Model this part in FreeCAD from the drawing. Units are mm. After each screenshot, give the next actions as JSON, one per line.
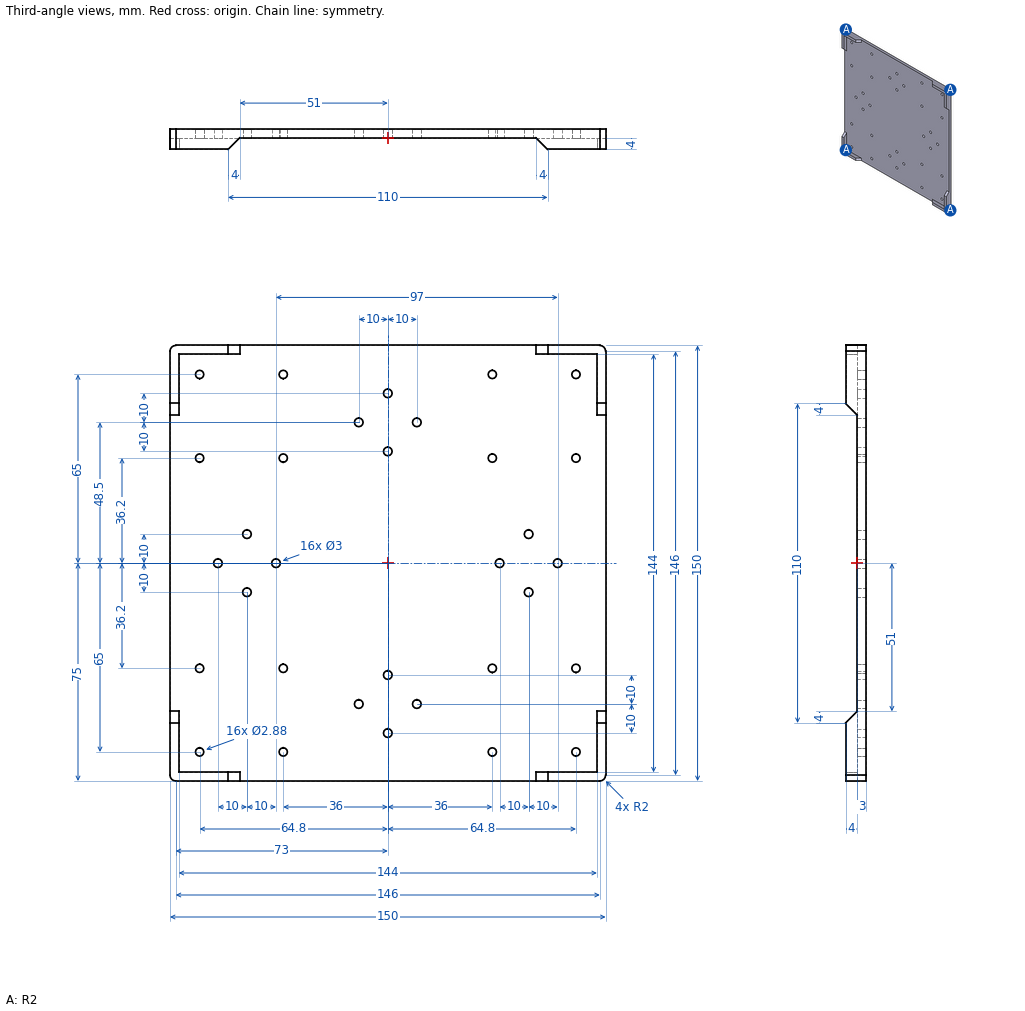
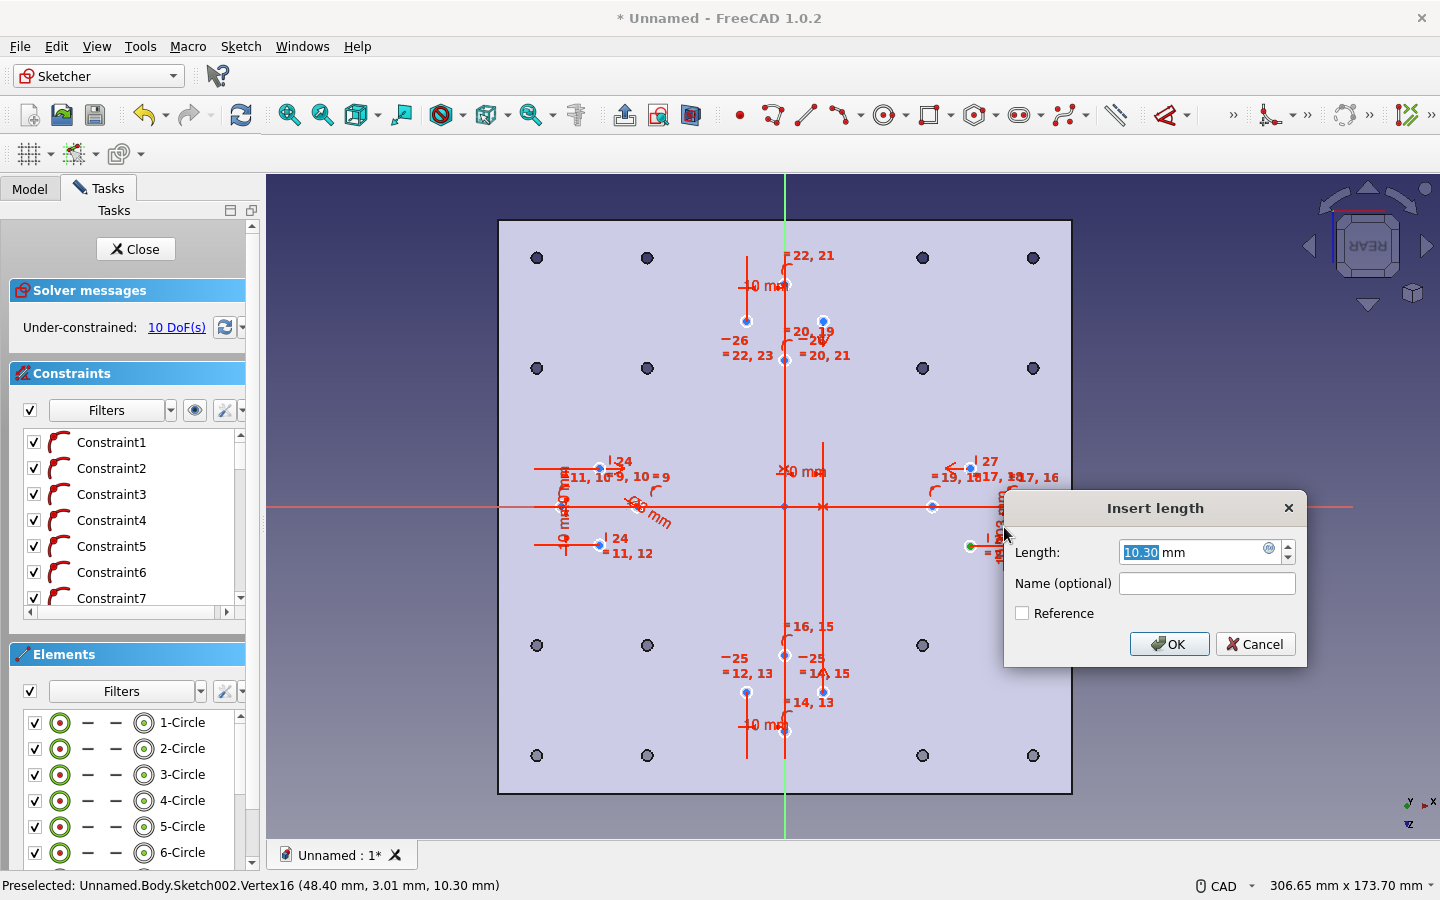
{"action": "type", "text": "10"}
{"action": "key", "text": "Return"}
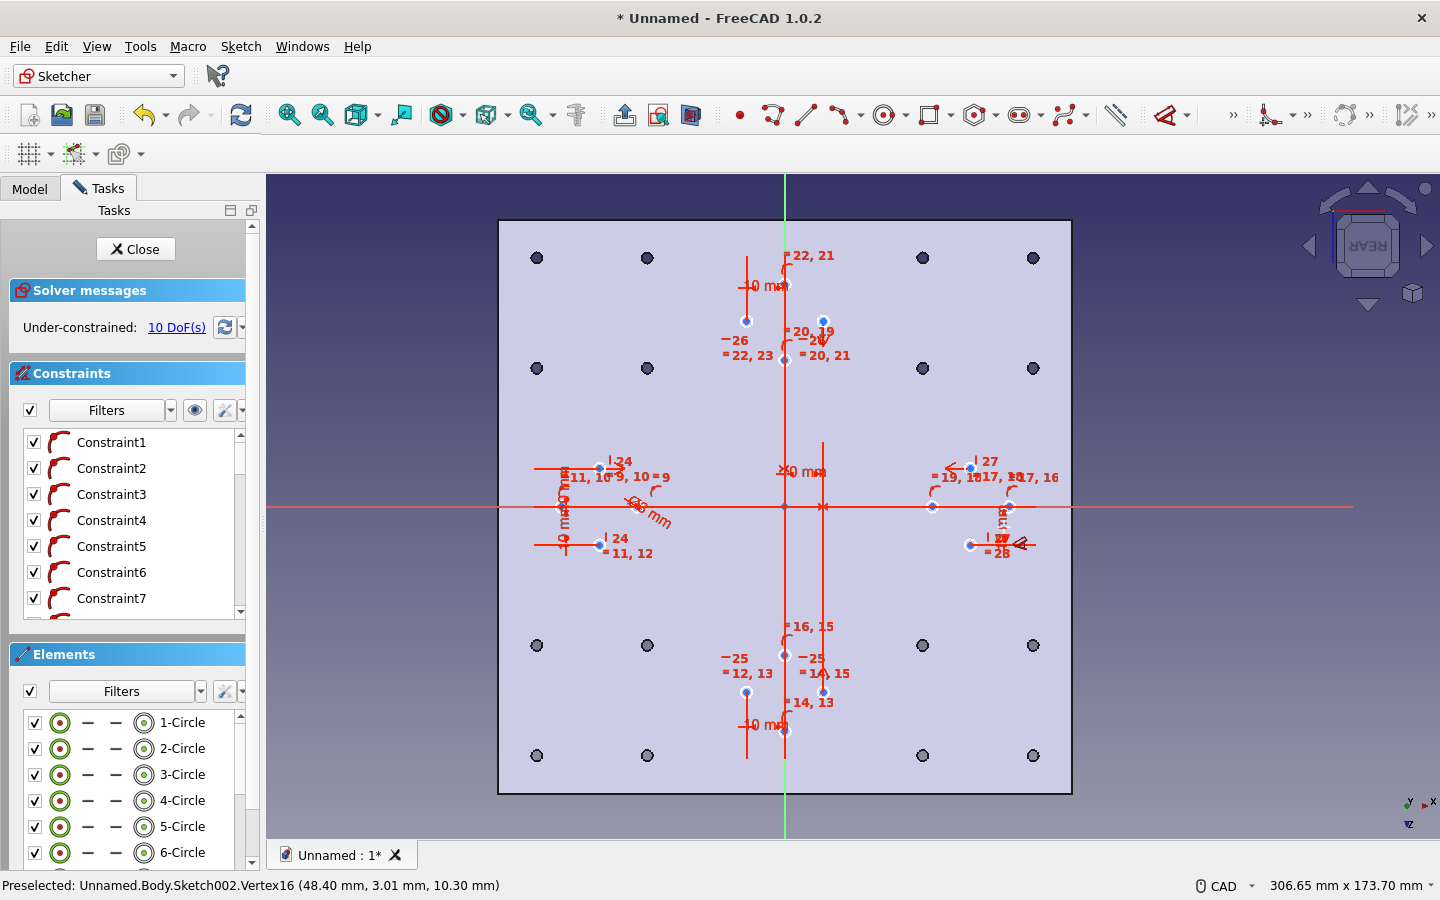
{"action": "left_click", "coordinate": [637, 507]}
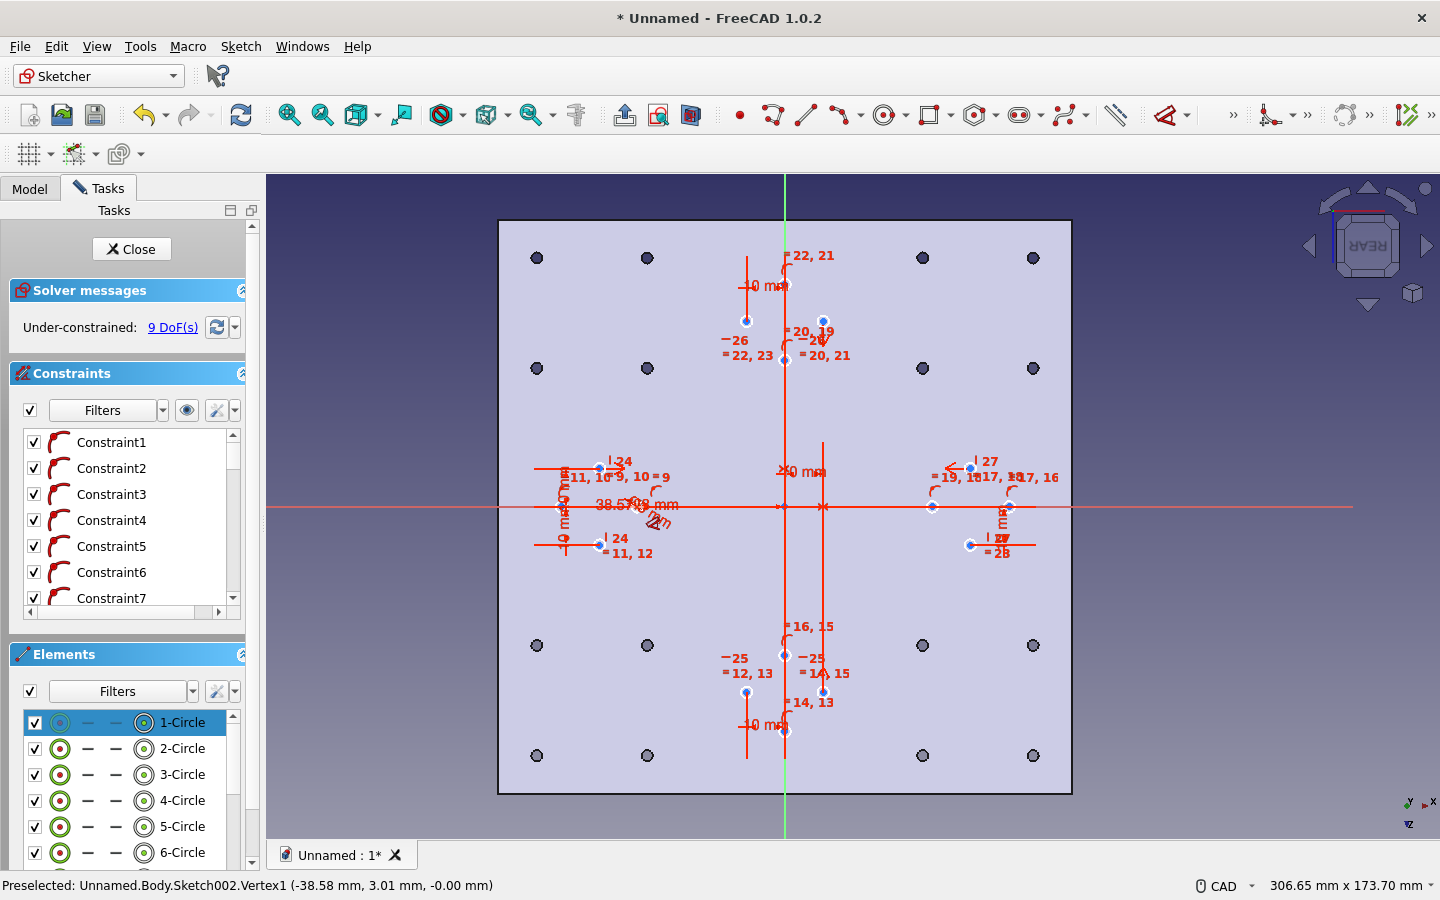
{"action": "left_click", "coordinate": [600, 469]}
{"action": "left_click", "coordinate": [618, 435]}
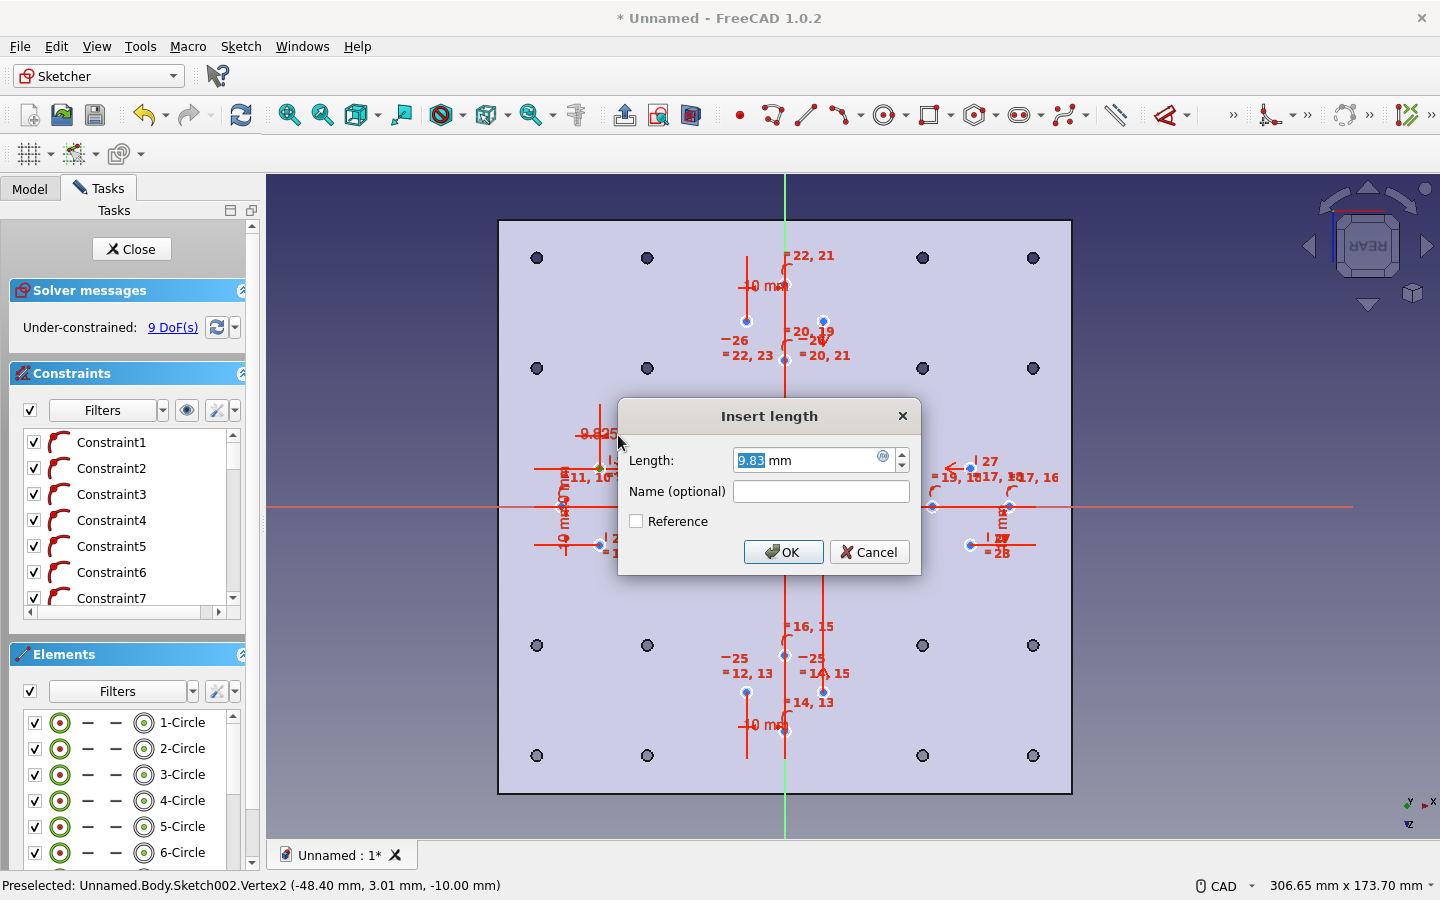
{"action": "type", "text": "10"}
{"action": "key", "text": "Return"}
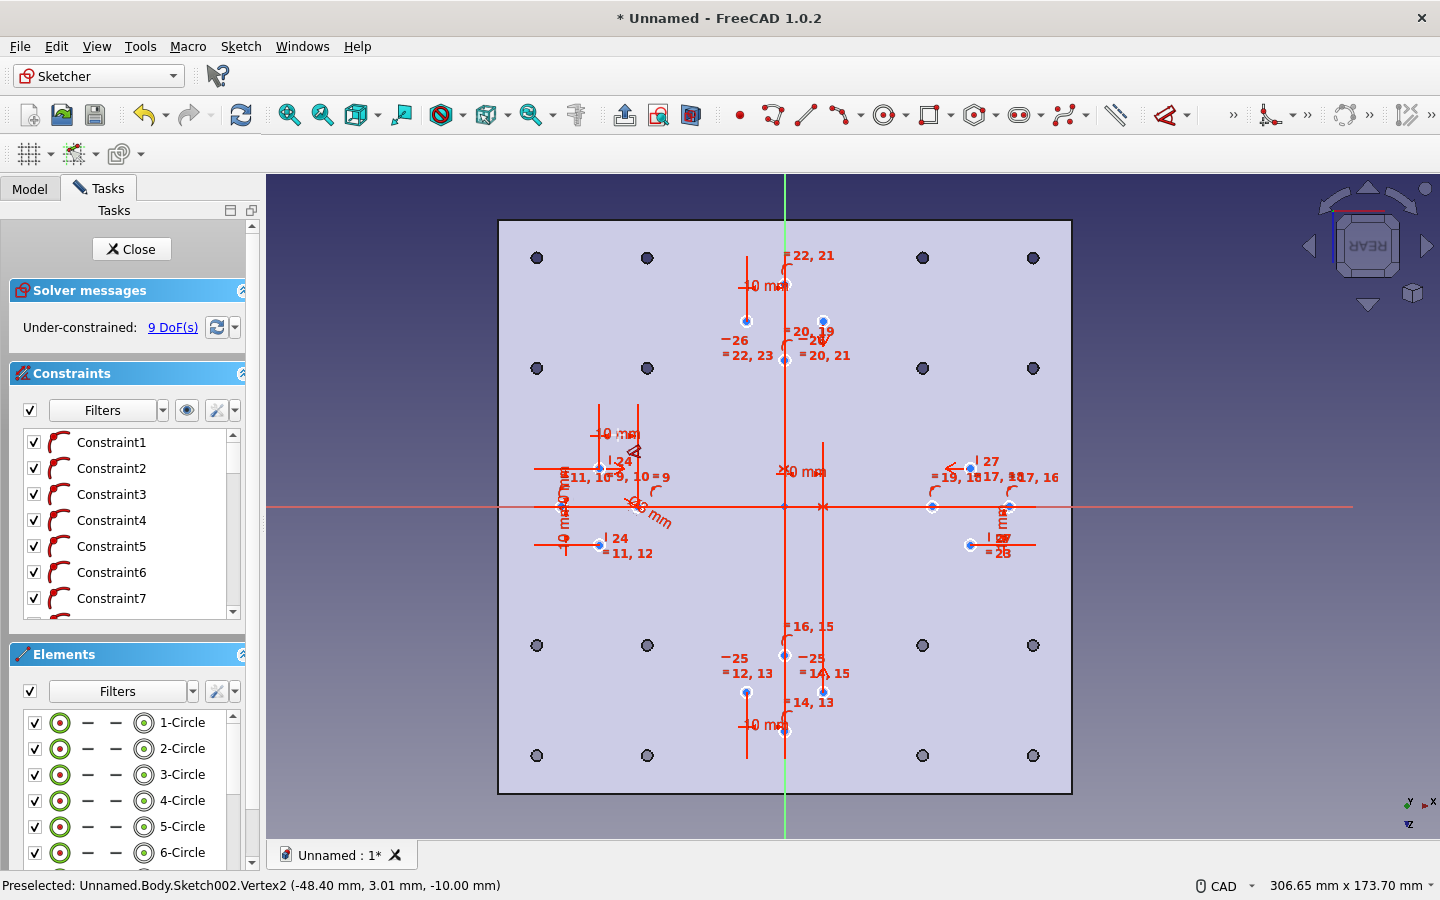
{"action": "left_click", "coordinate": [599, 469]}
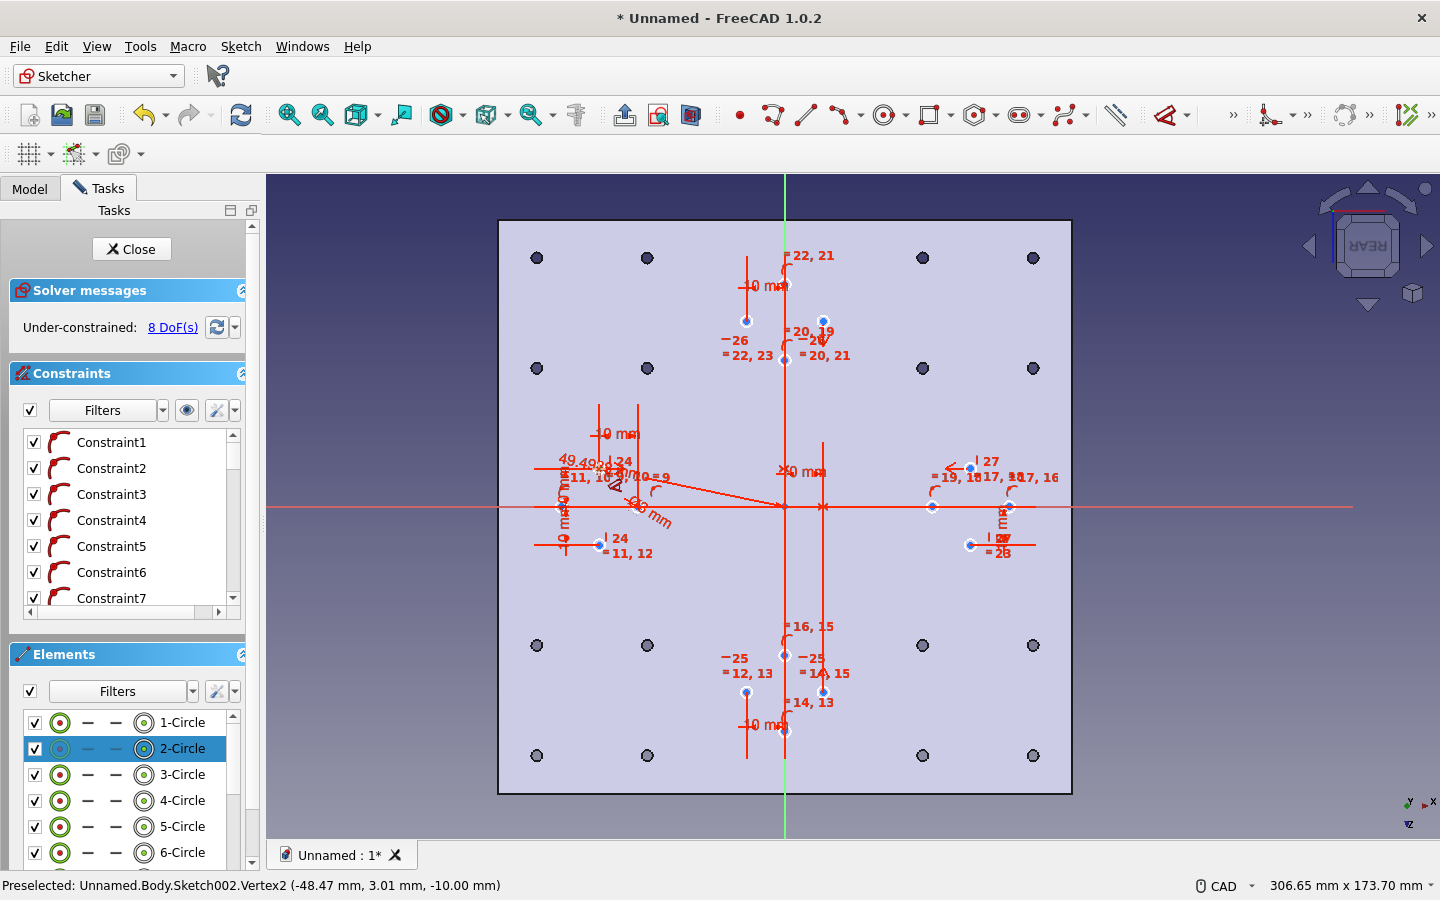
{"action": "left_click", "coordinate": [561, 507]}
{"action": "left_click", "coordinate": [580, 411]}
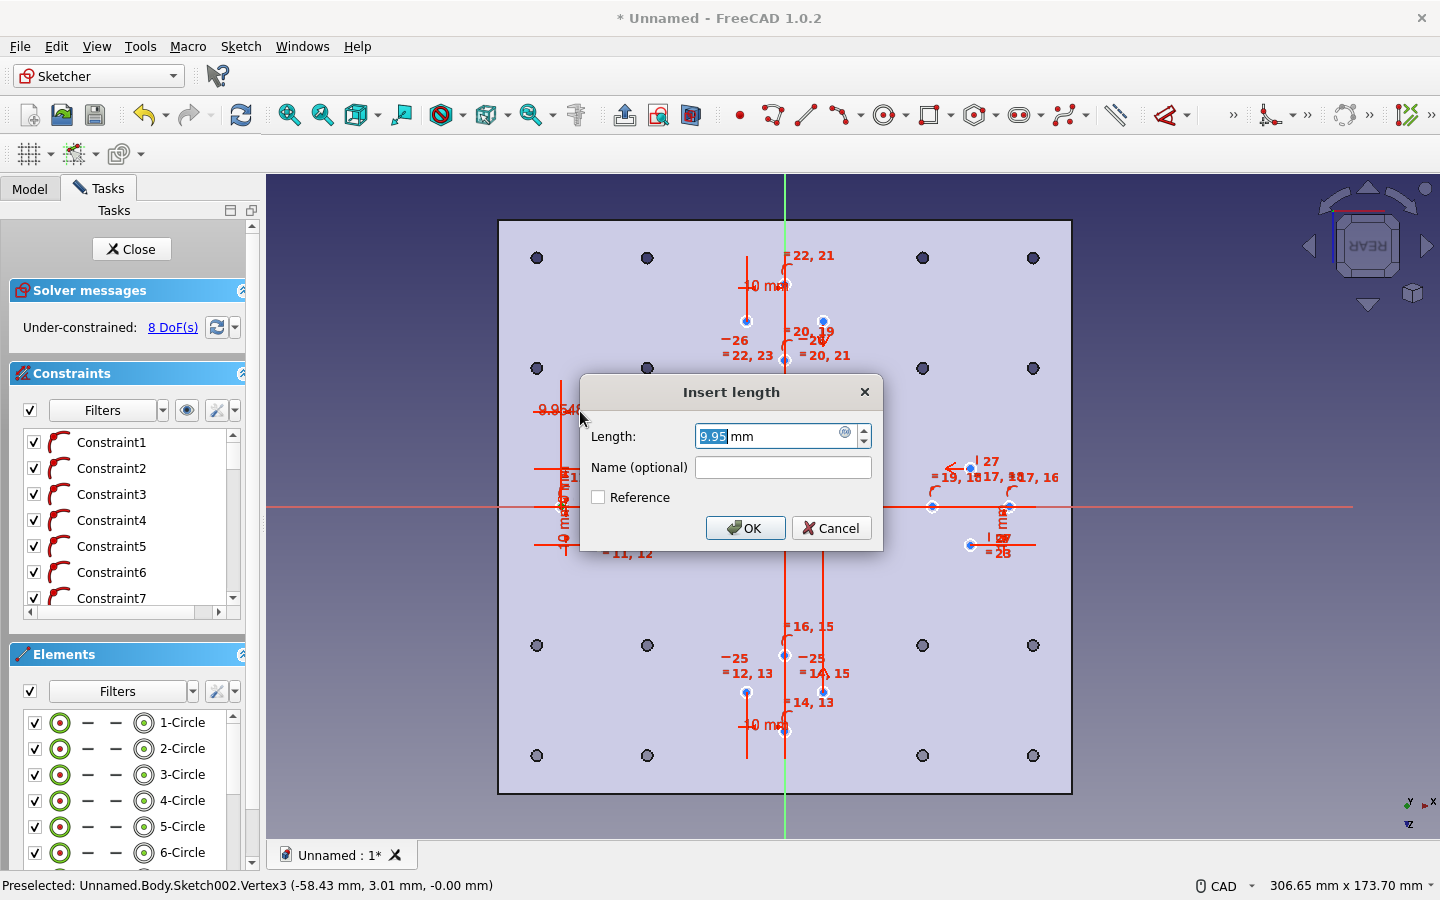
{"action": "type", "text": "10"}
{"action": "key", "text": "Return"}